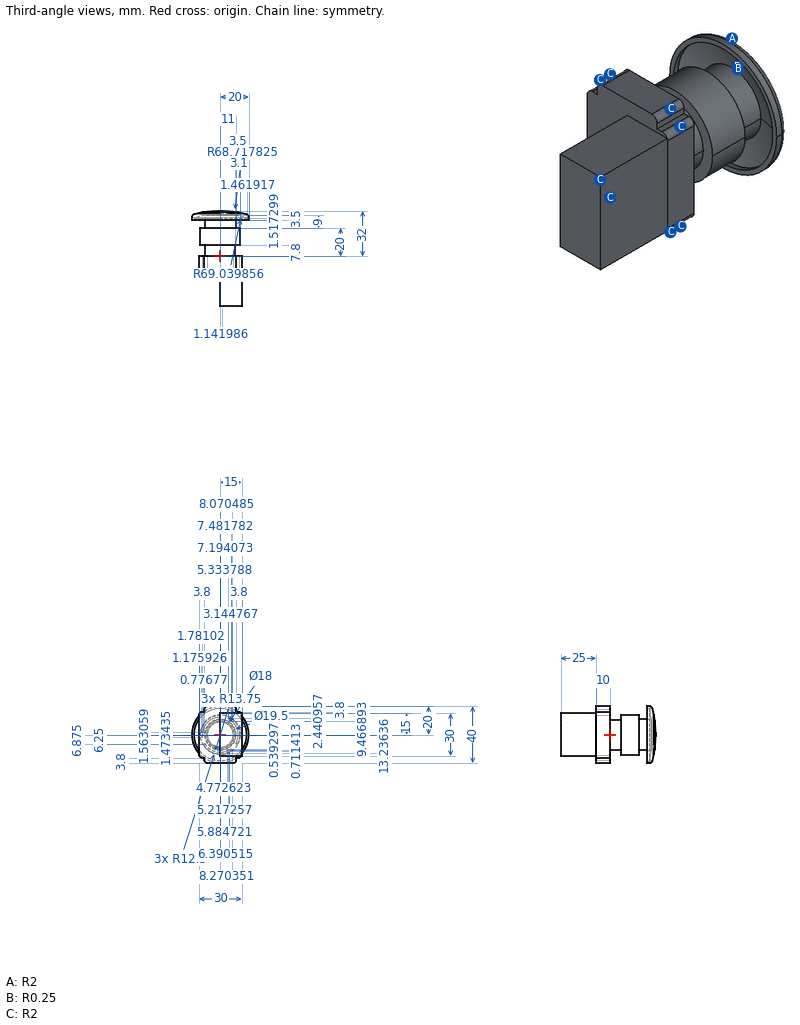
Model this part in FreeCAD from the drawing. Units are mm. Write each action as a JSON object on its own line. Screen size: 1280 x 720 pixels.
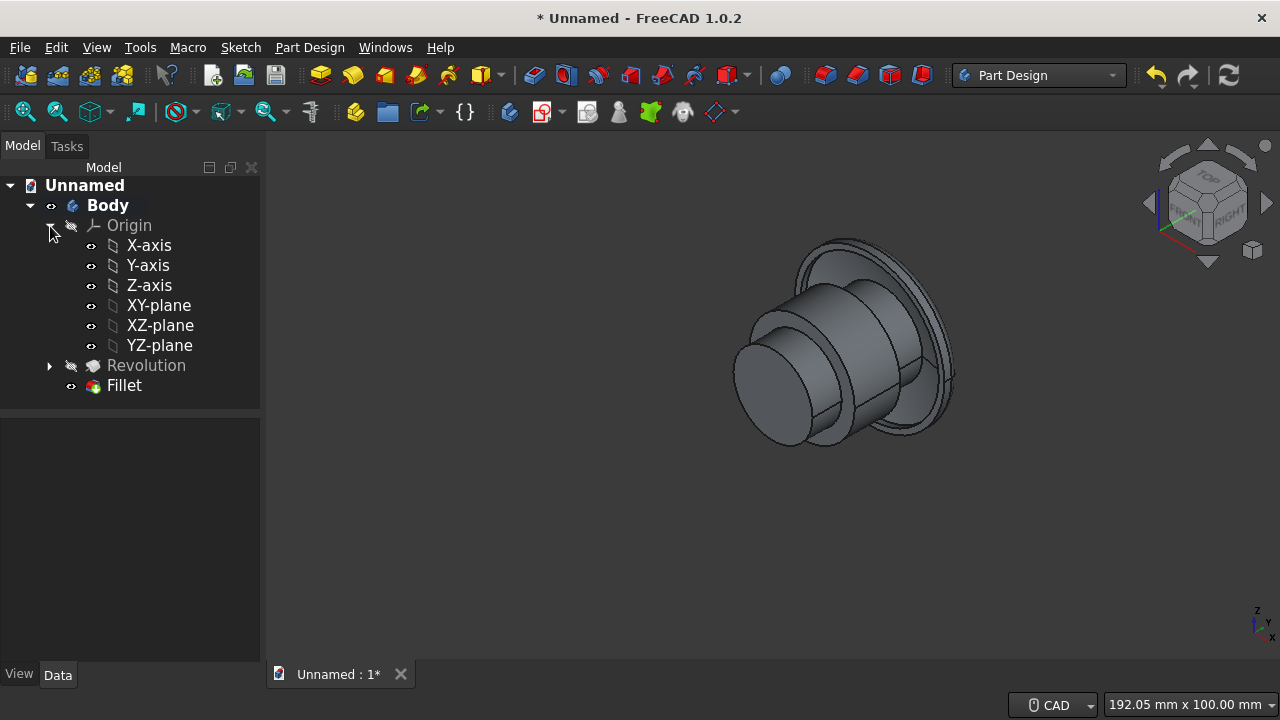
{"action": "left_click", "coordinate": [136, 326]}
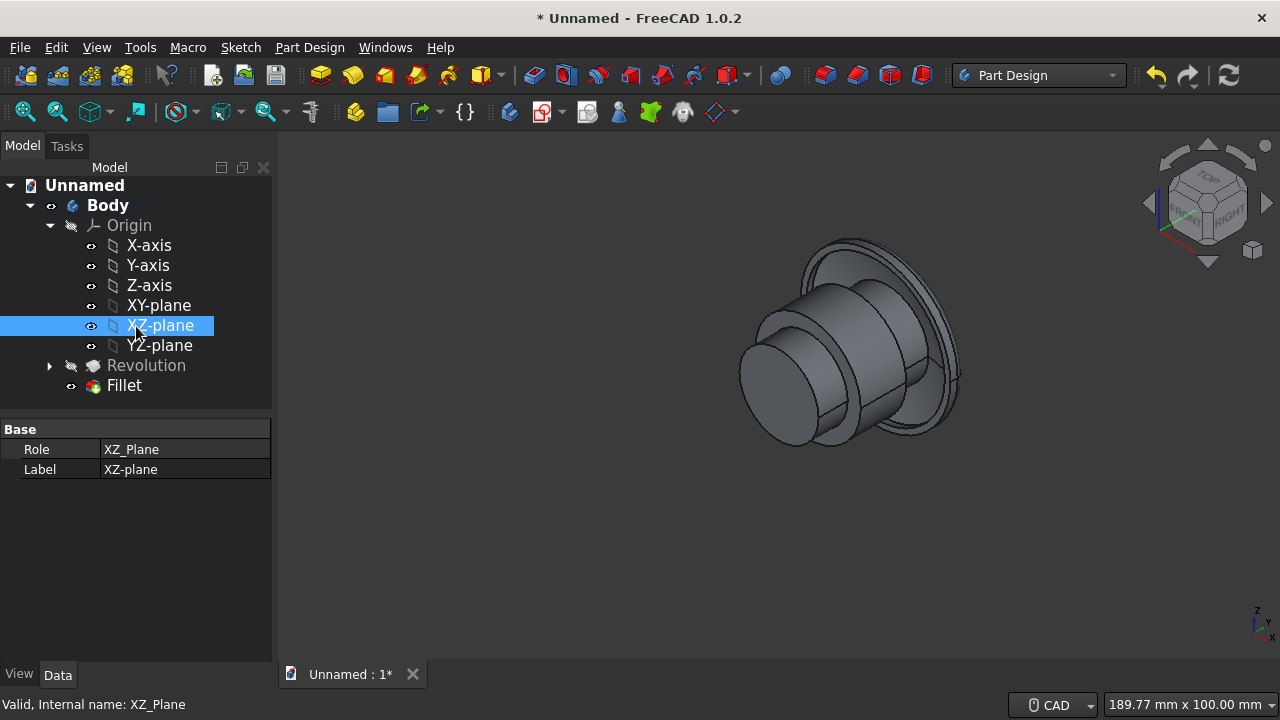
{"action": "left_click", "coordinate": [716, 112]}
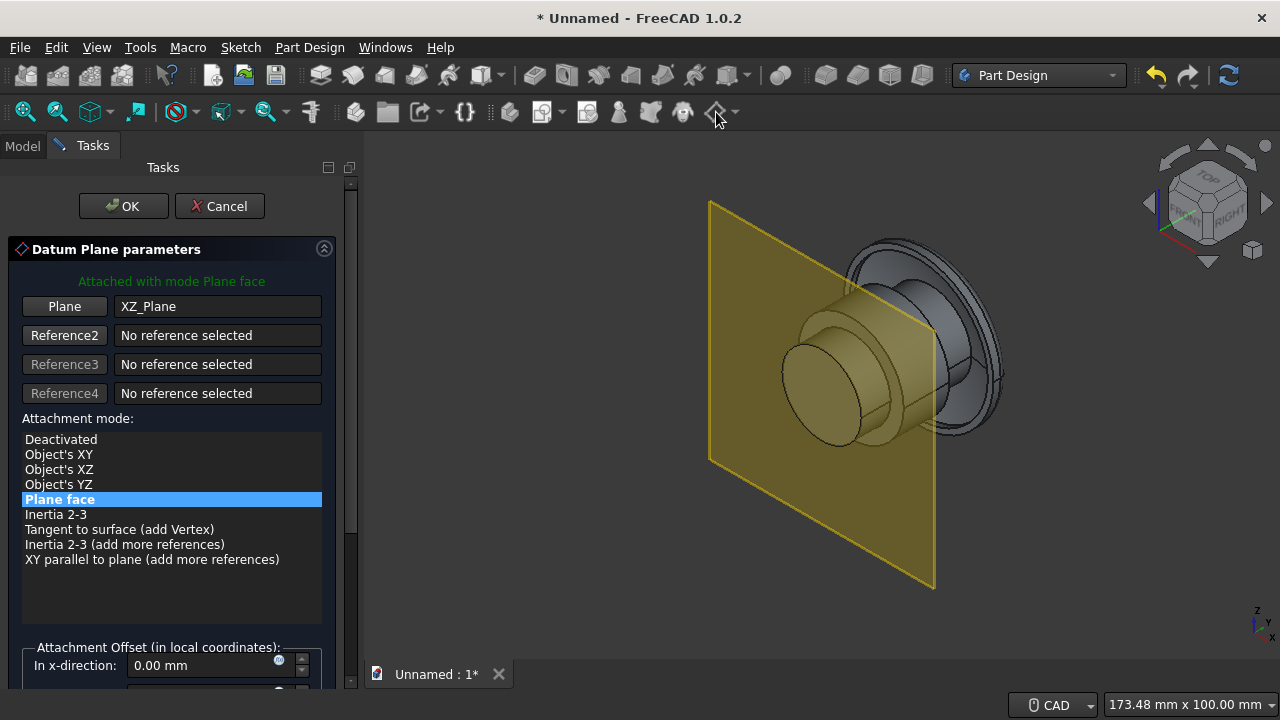
{"action": "scroll", "coordinate": [351, 432], "scroll_direction": "down", "scroll_amount": 2}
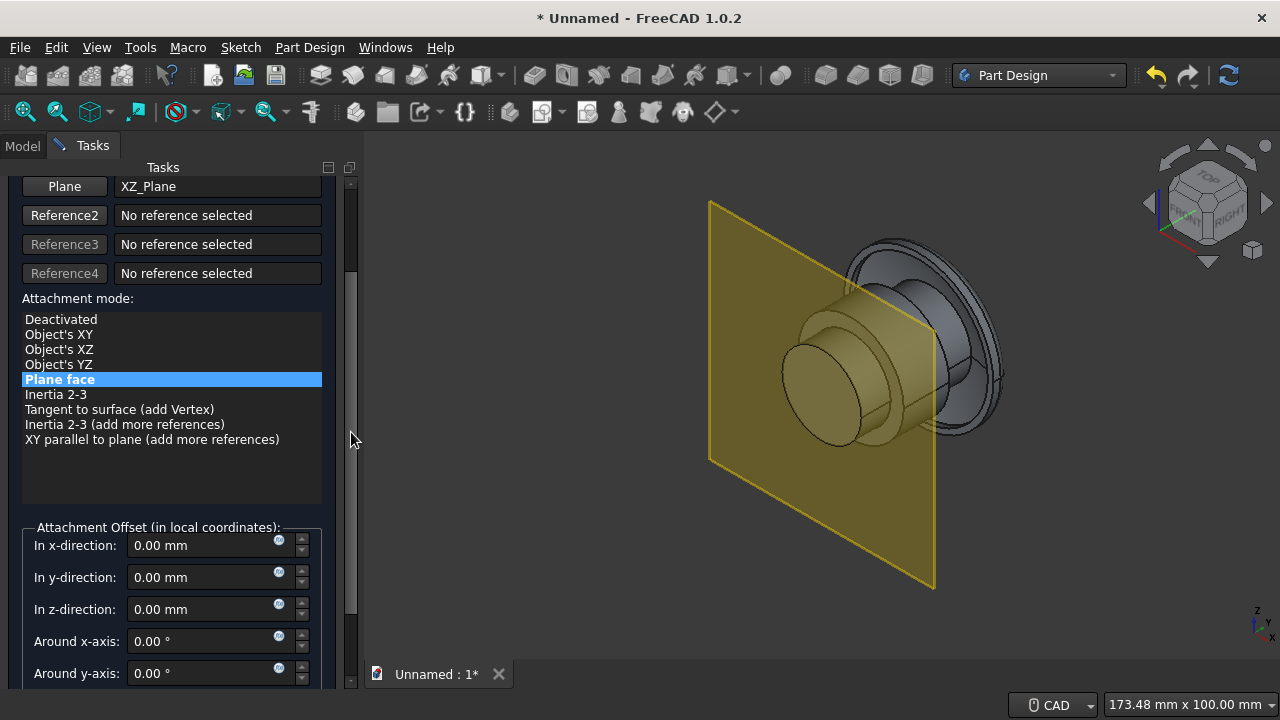
{"action": "triple_click", "coordinate": [210, 609]}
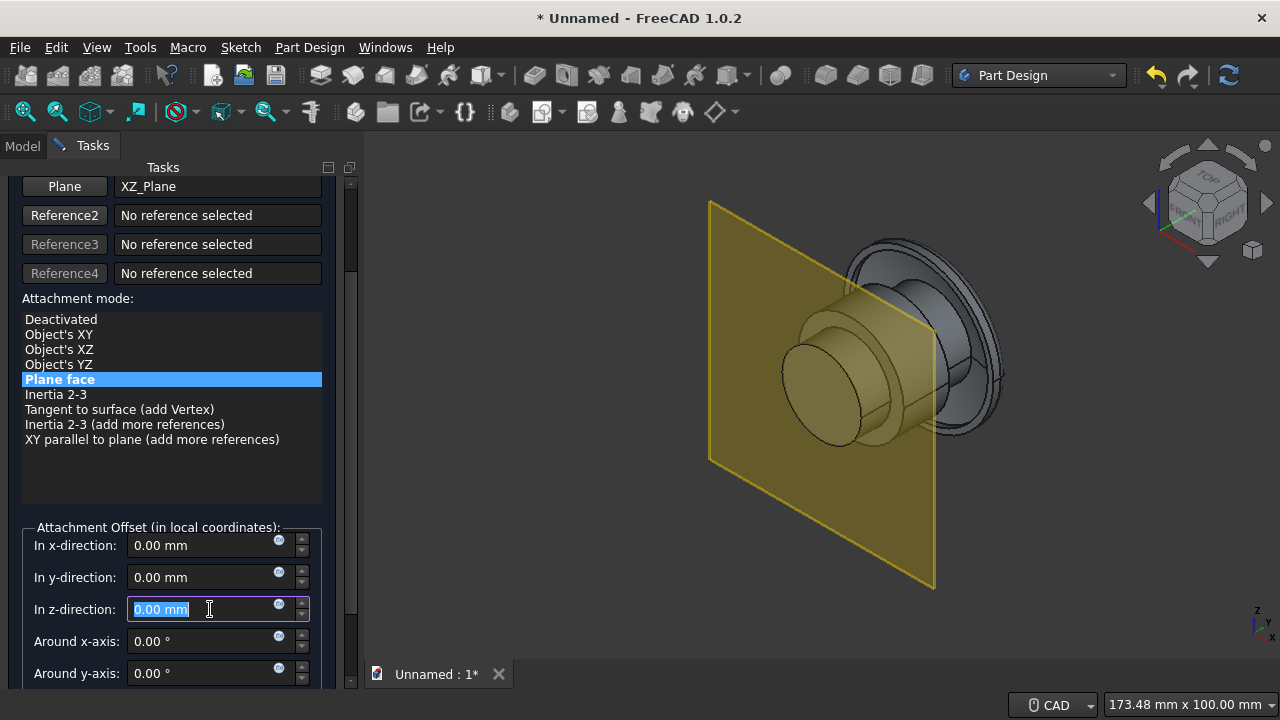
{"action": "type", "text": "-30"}
{"action": "key", "text": "Tab"}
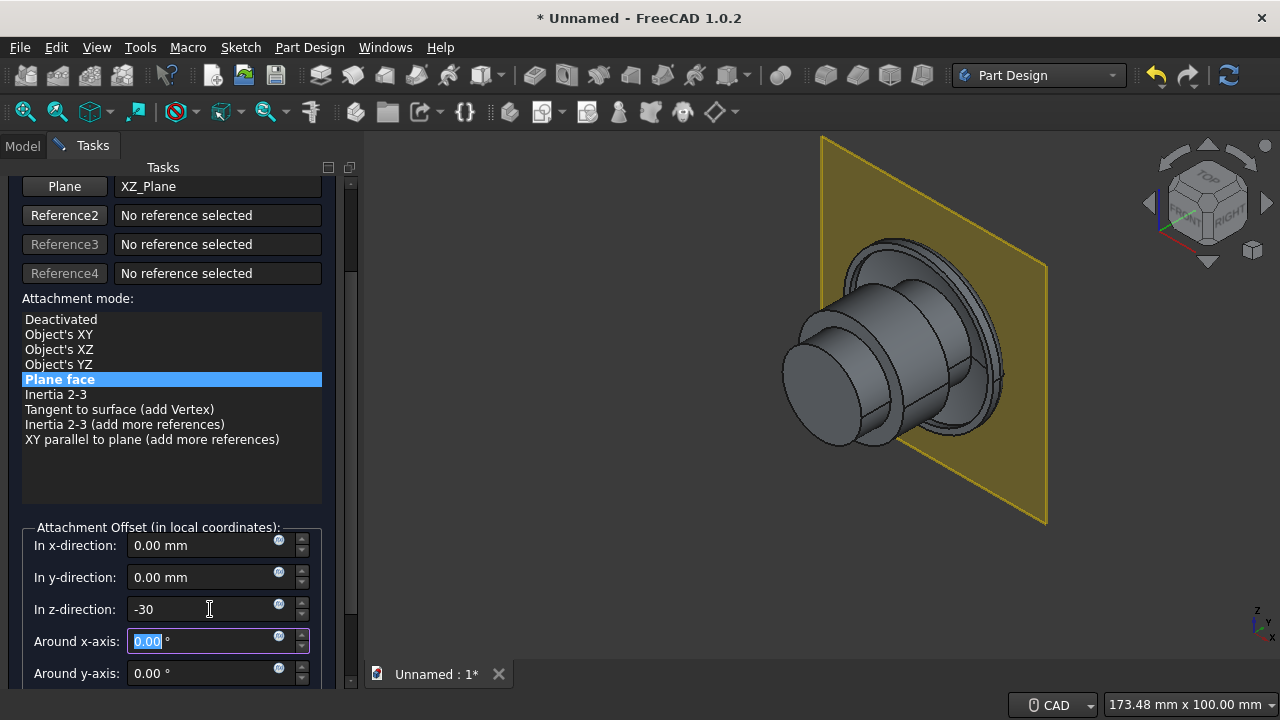
{"action": "scroll", "coordinate": [351, 432], "scroll_direction": "up", "scroll_amount": 3}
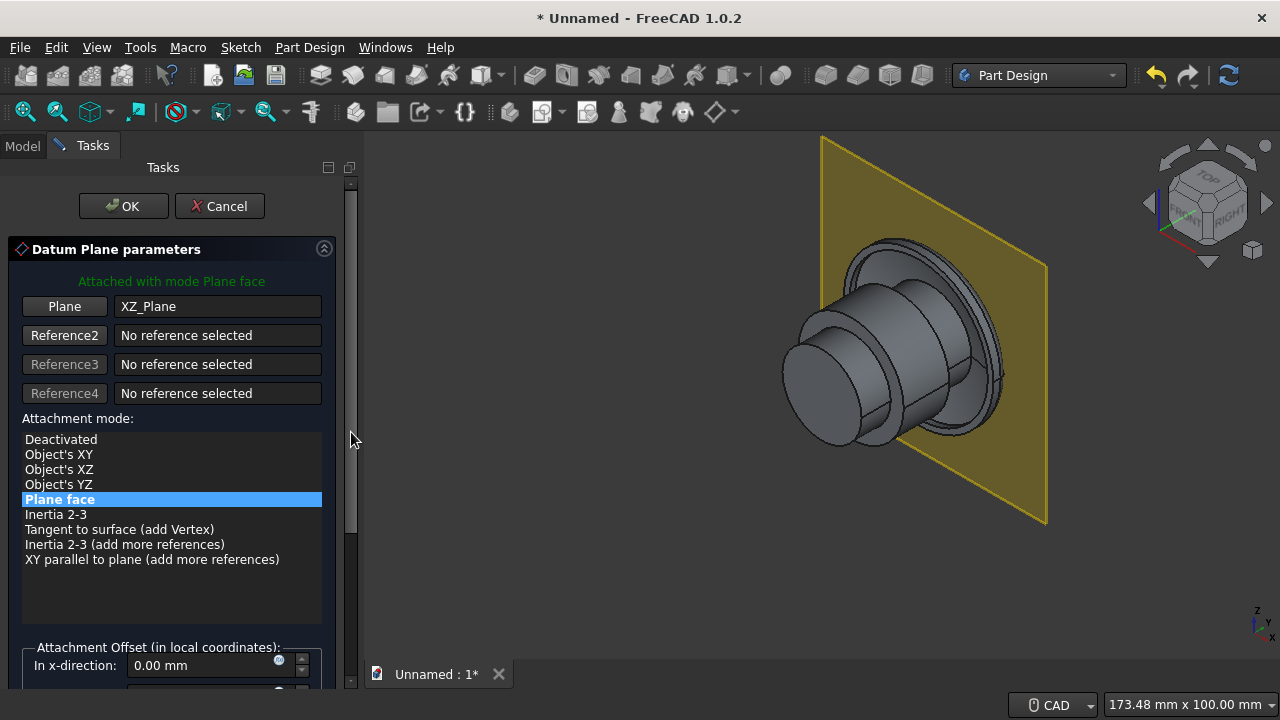
{"action": "left_click", "coordinate": [124, 206]}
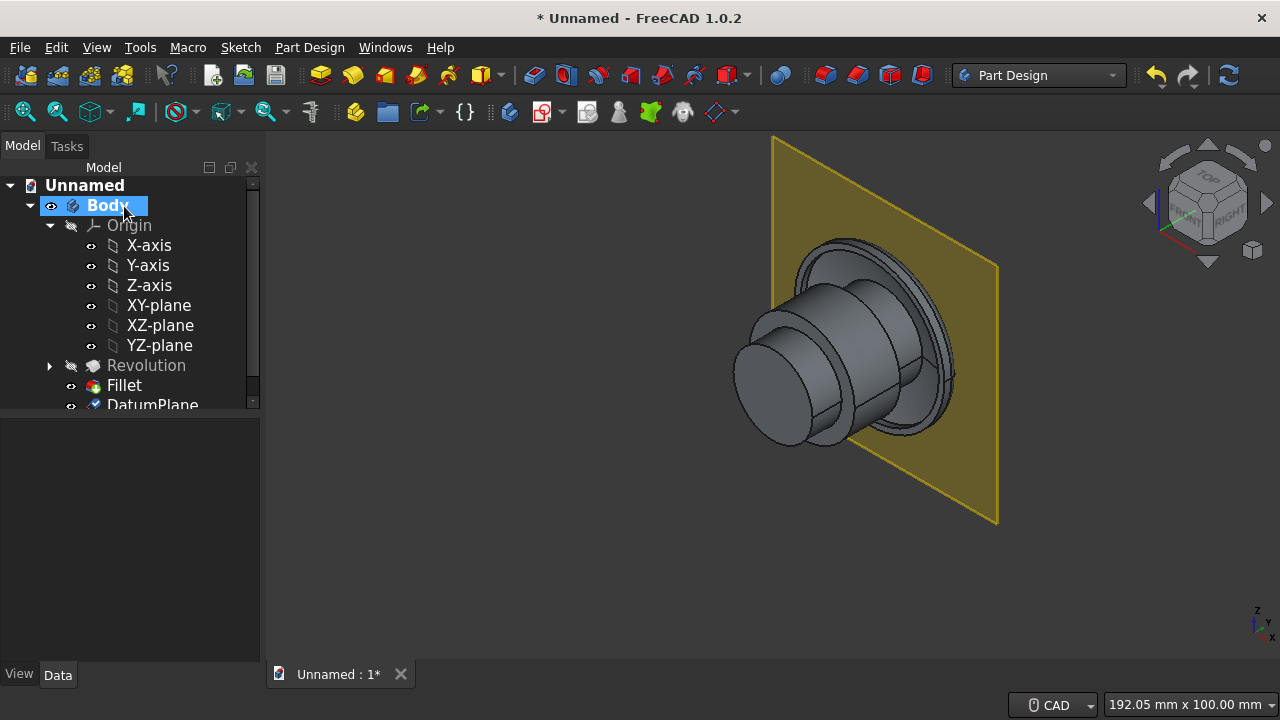
{"action": "left_click", "coordinate": [116, 406]}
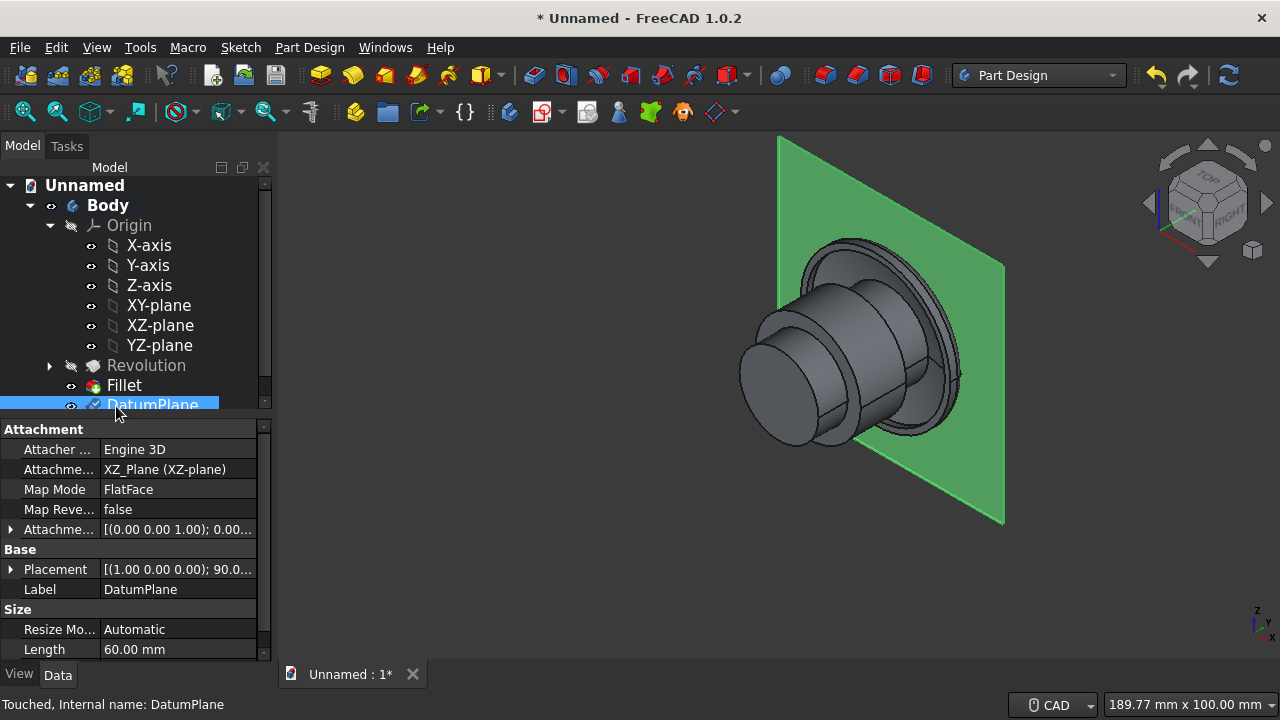
{"action": "left_click", "coordinate": [542, 112]}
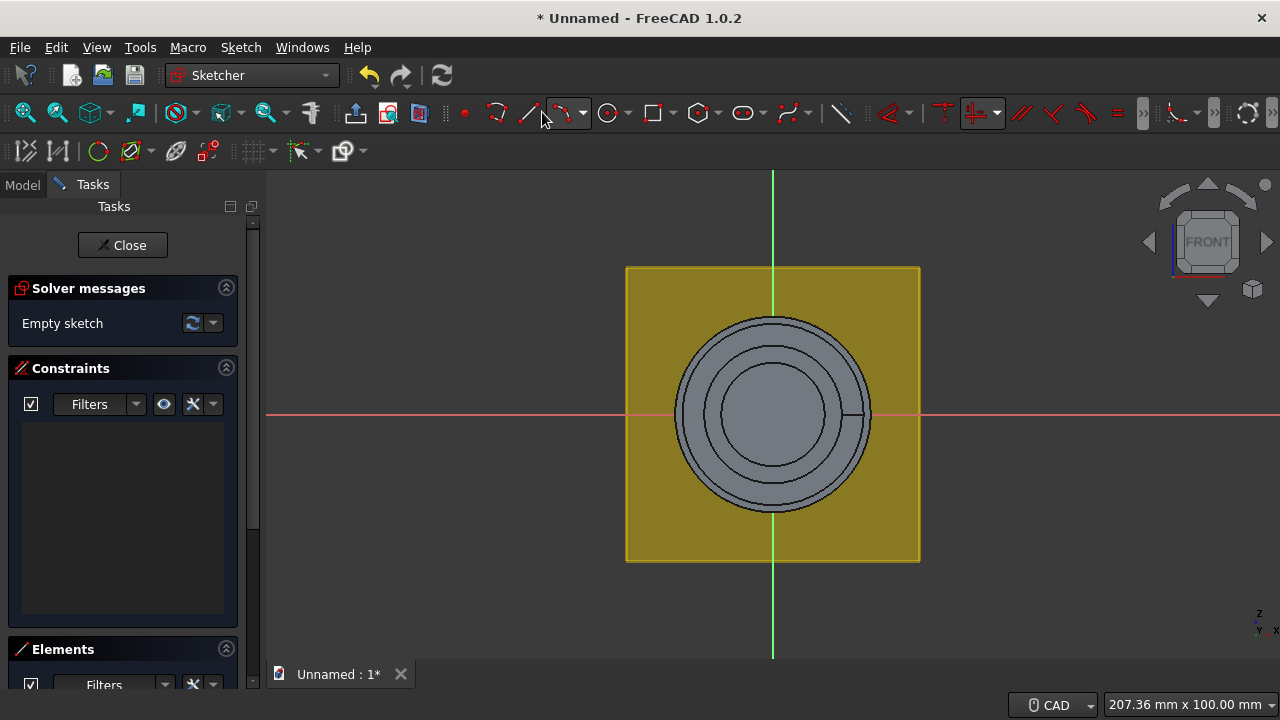
{"action": "left_click", "coordinate": [420, 114]}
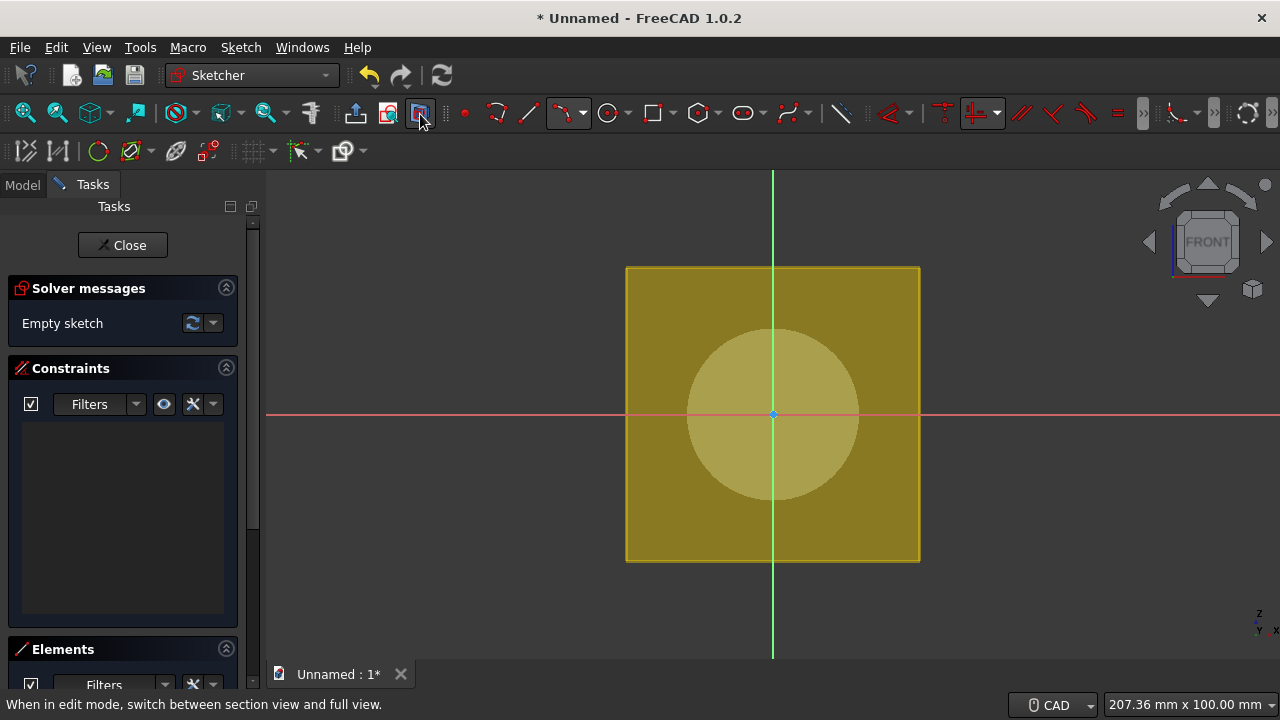
{"action": "scroll", "coordinate": [803, 414], "scroll_direction": "up", "scroll_amount": 6}